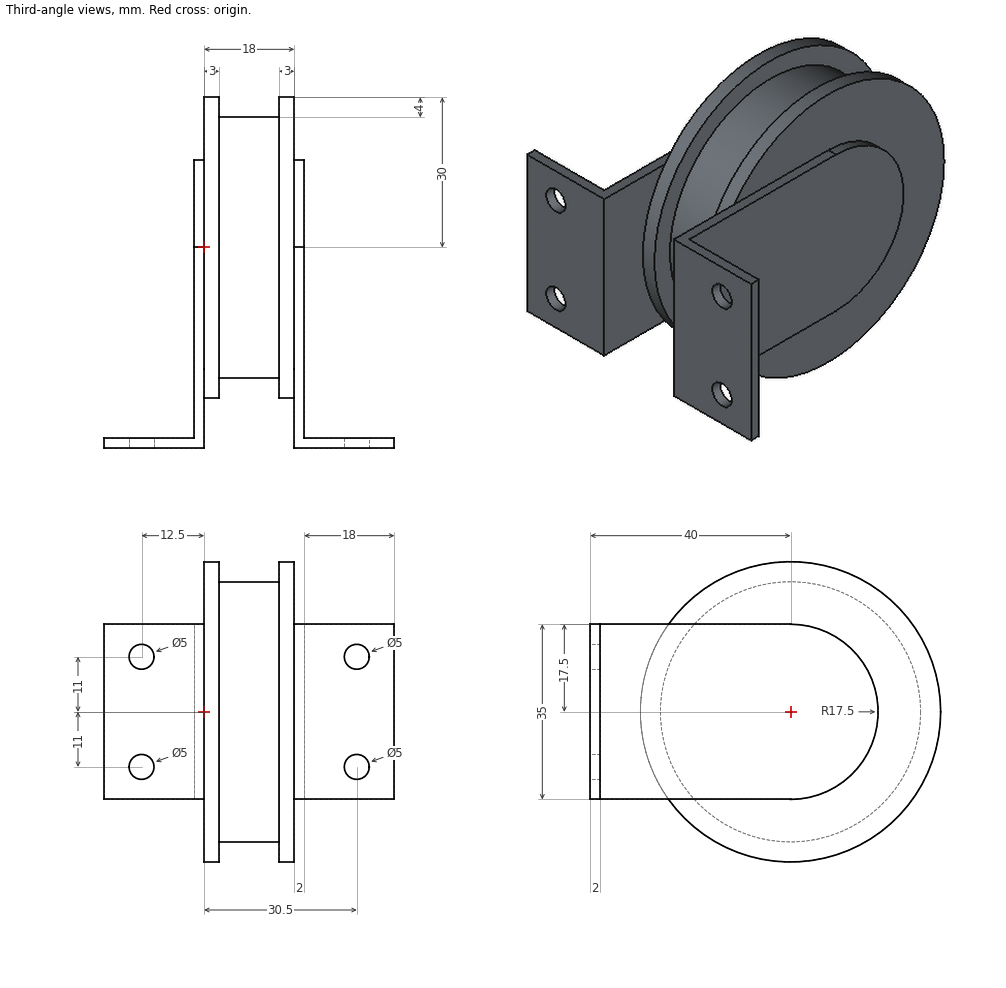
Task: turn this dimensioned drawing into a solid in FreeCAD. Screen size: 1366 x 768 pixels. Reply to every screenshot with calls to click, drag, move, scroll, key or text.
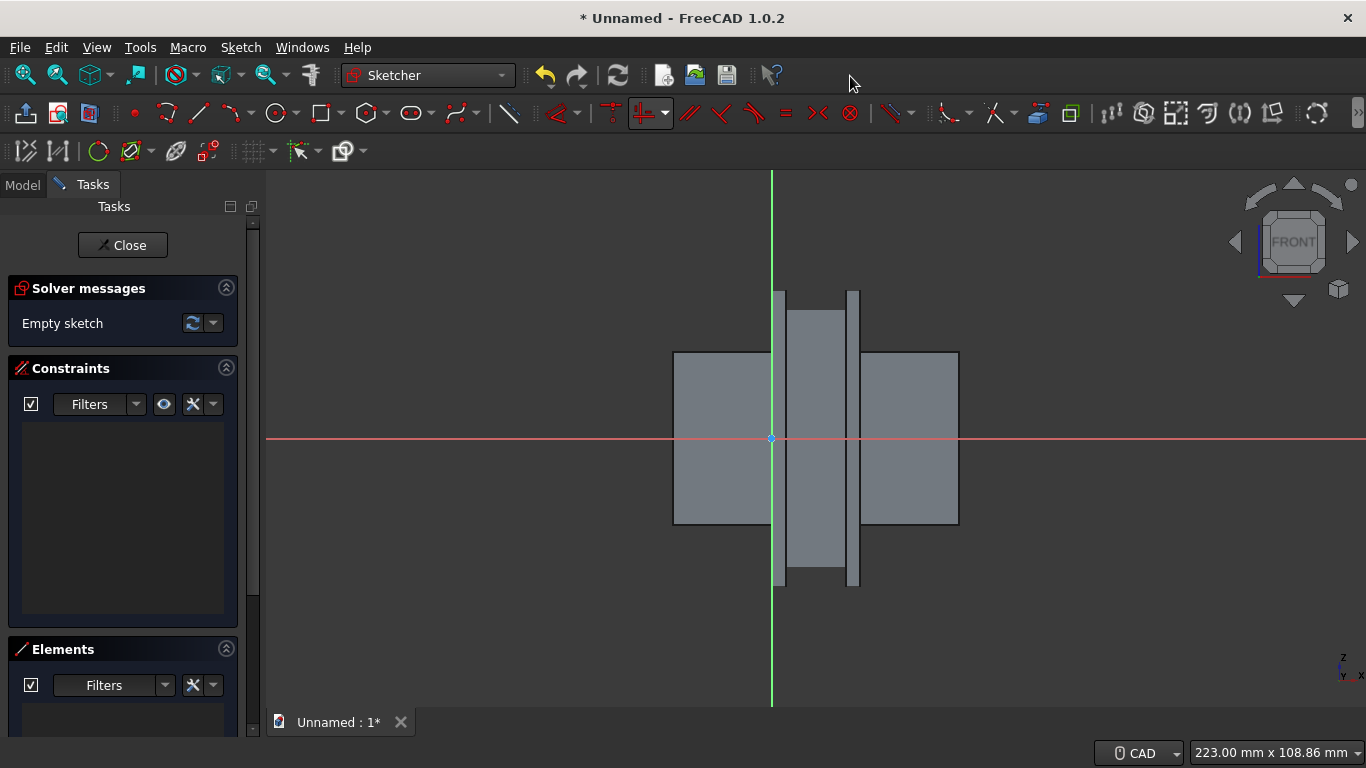
scroll(707, 380, up, 13)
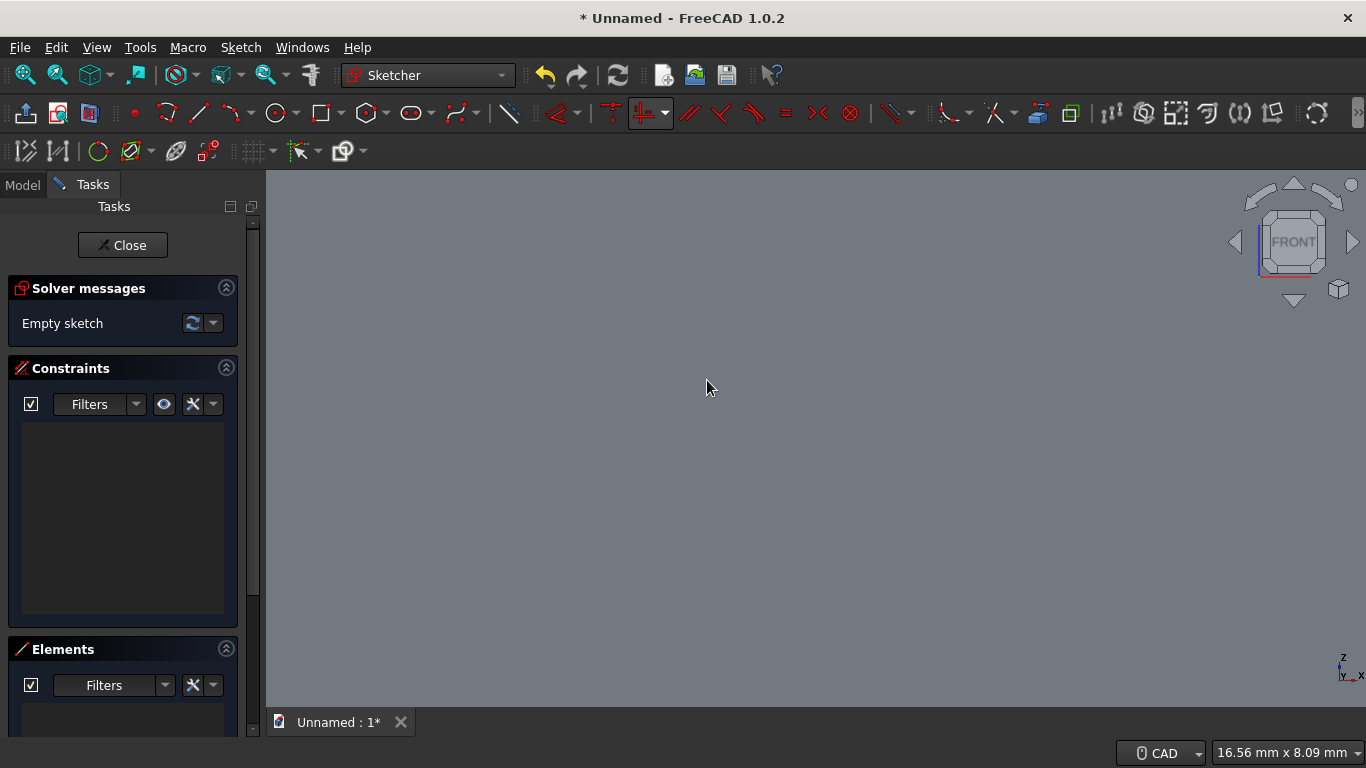
click(276, 114)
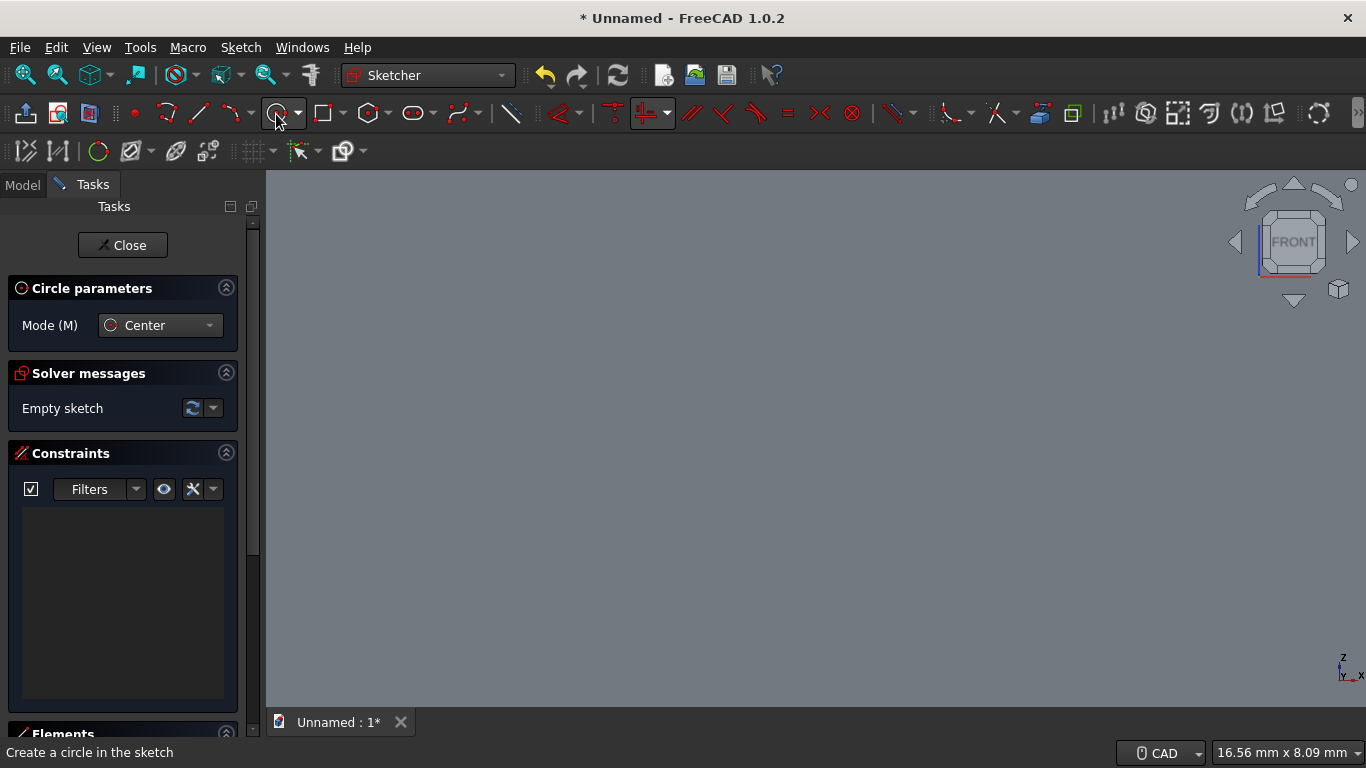
click(742, 432)
click(859, 315)
key(Escape)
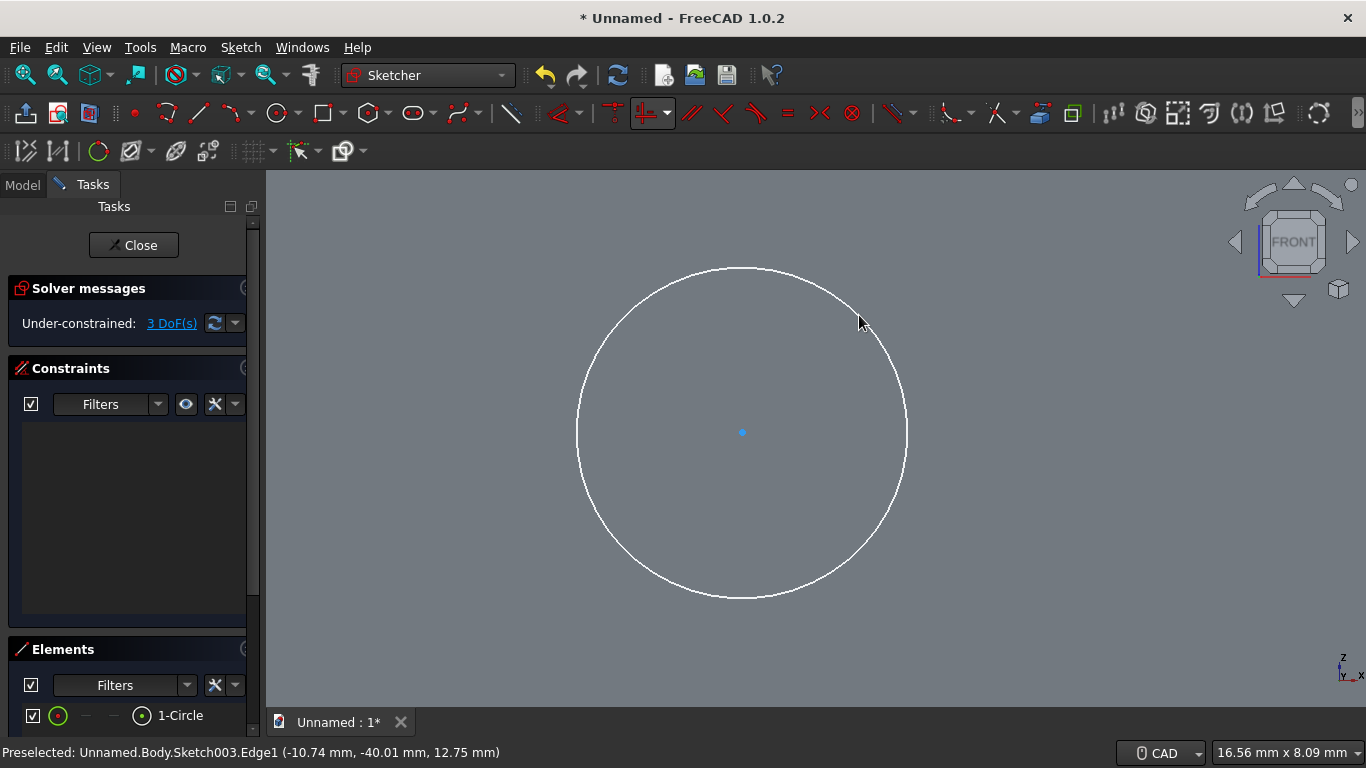
key(d)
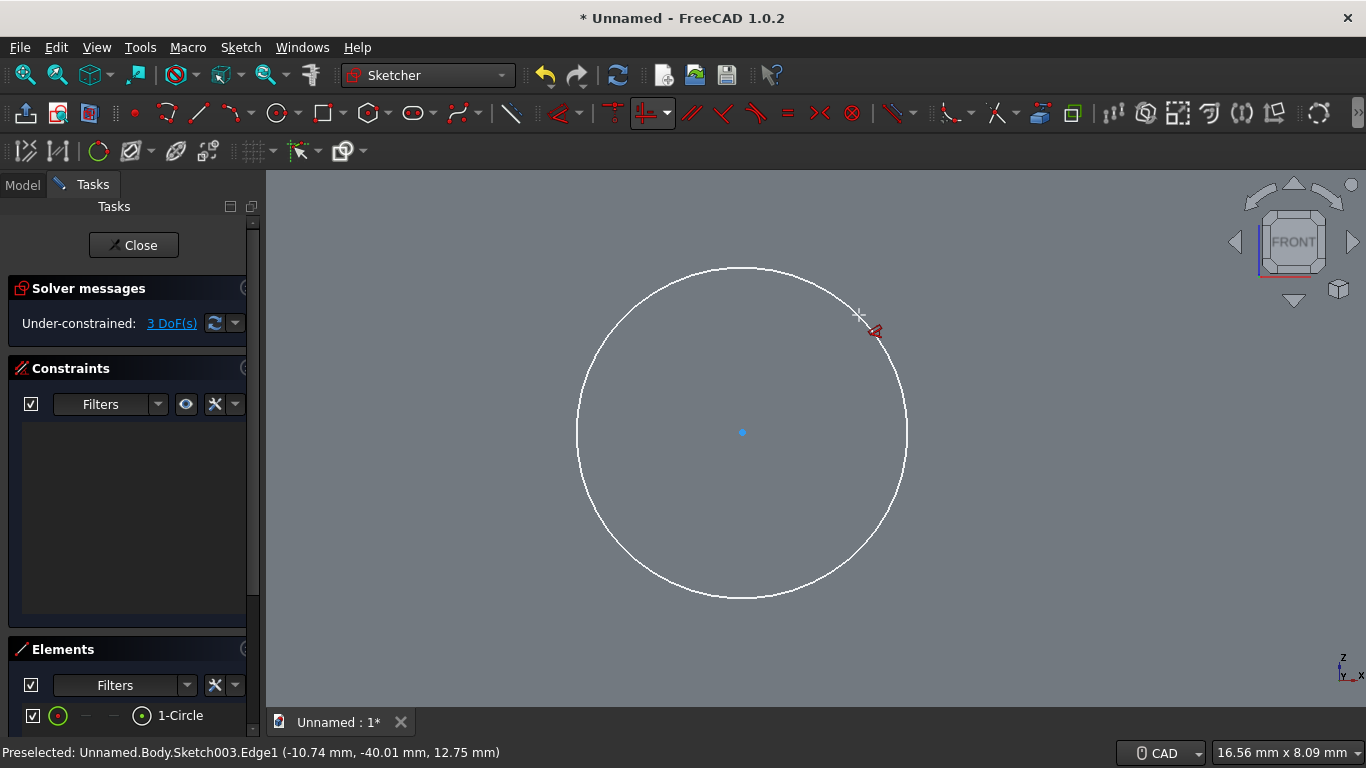
click(859, 316)
click(882, 293)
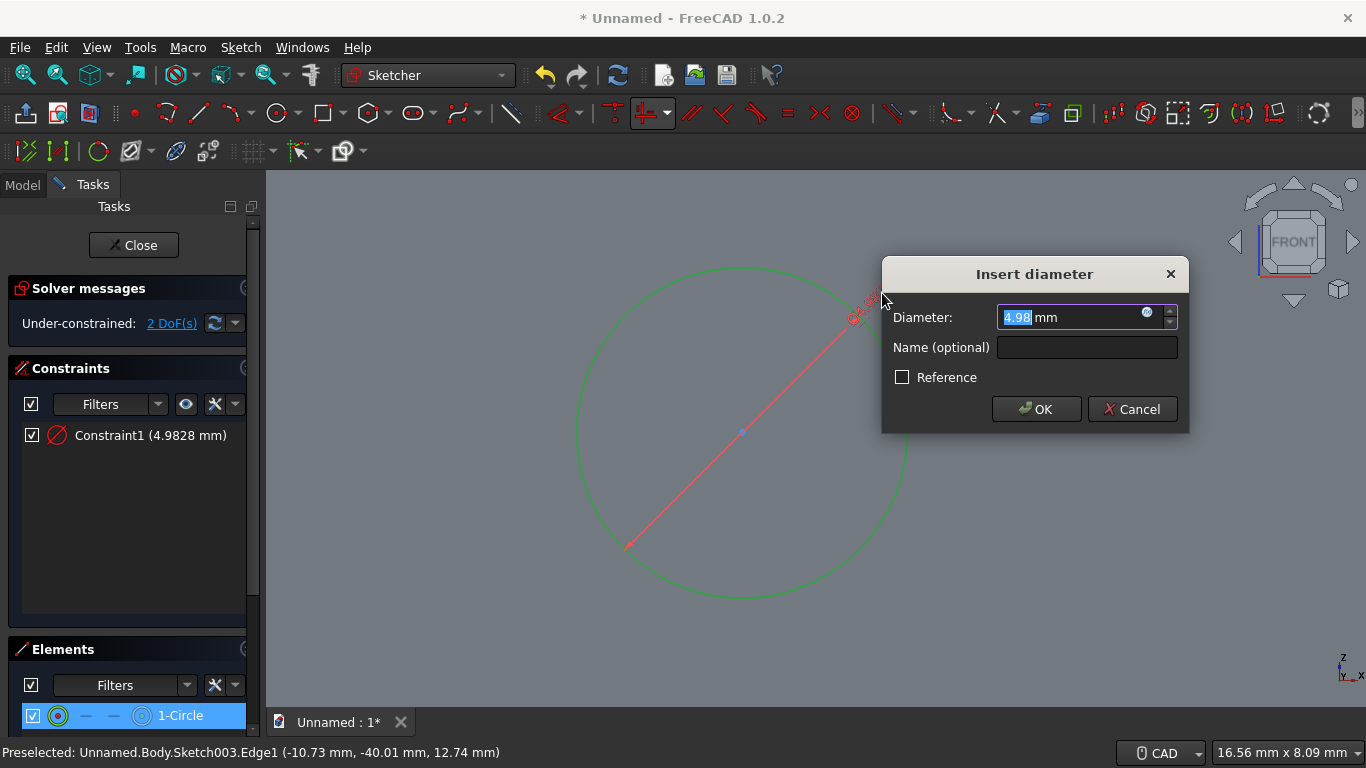
text(5)
key(Return)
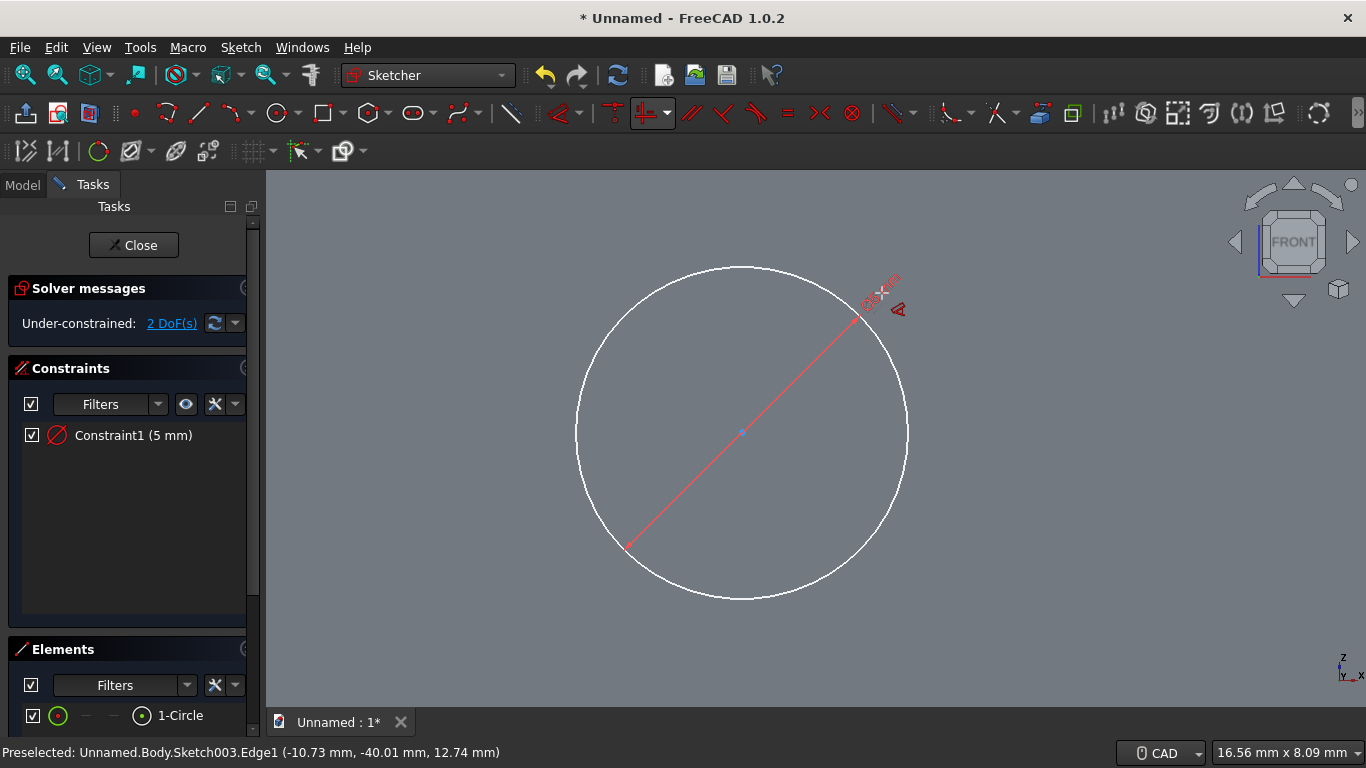
click(742, 433)
click(708, 556)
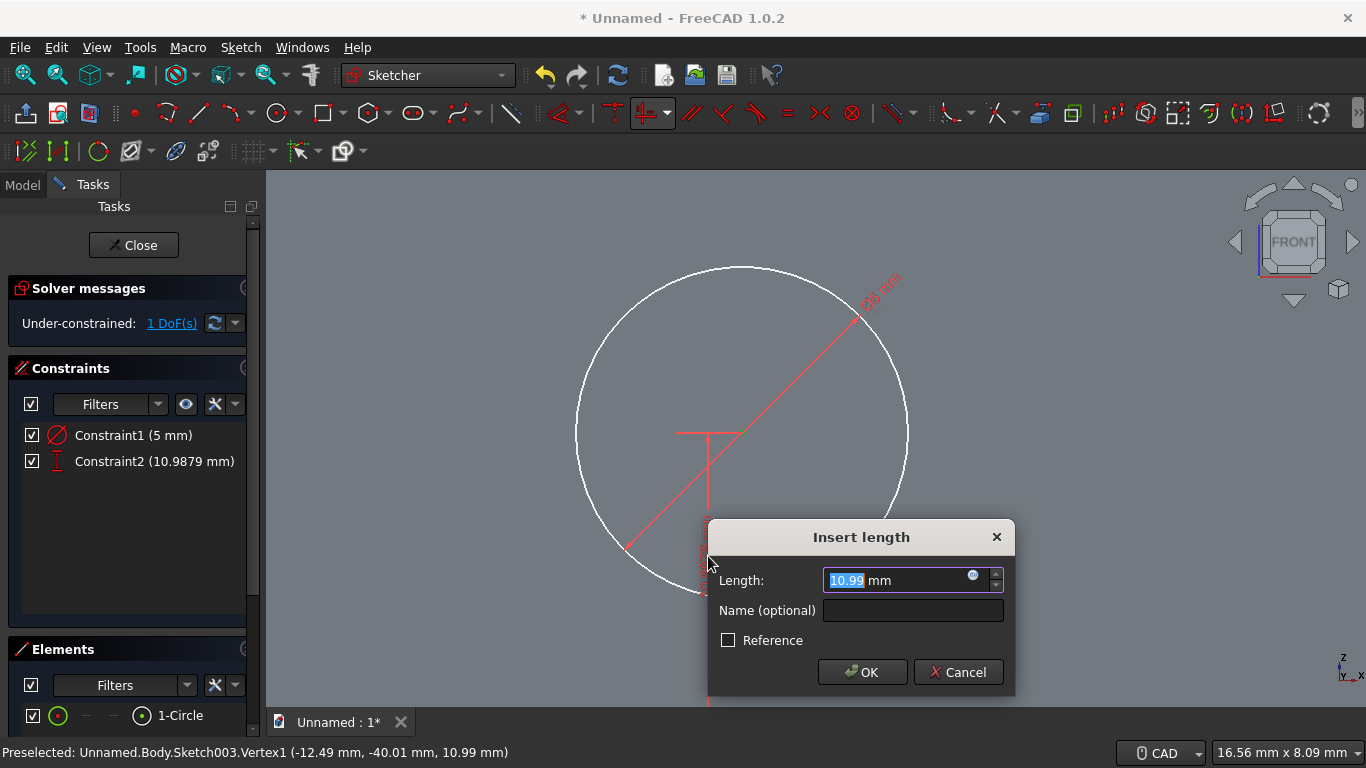
text(11)
key(Return)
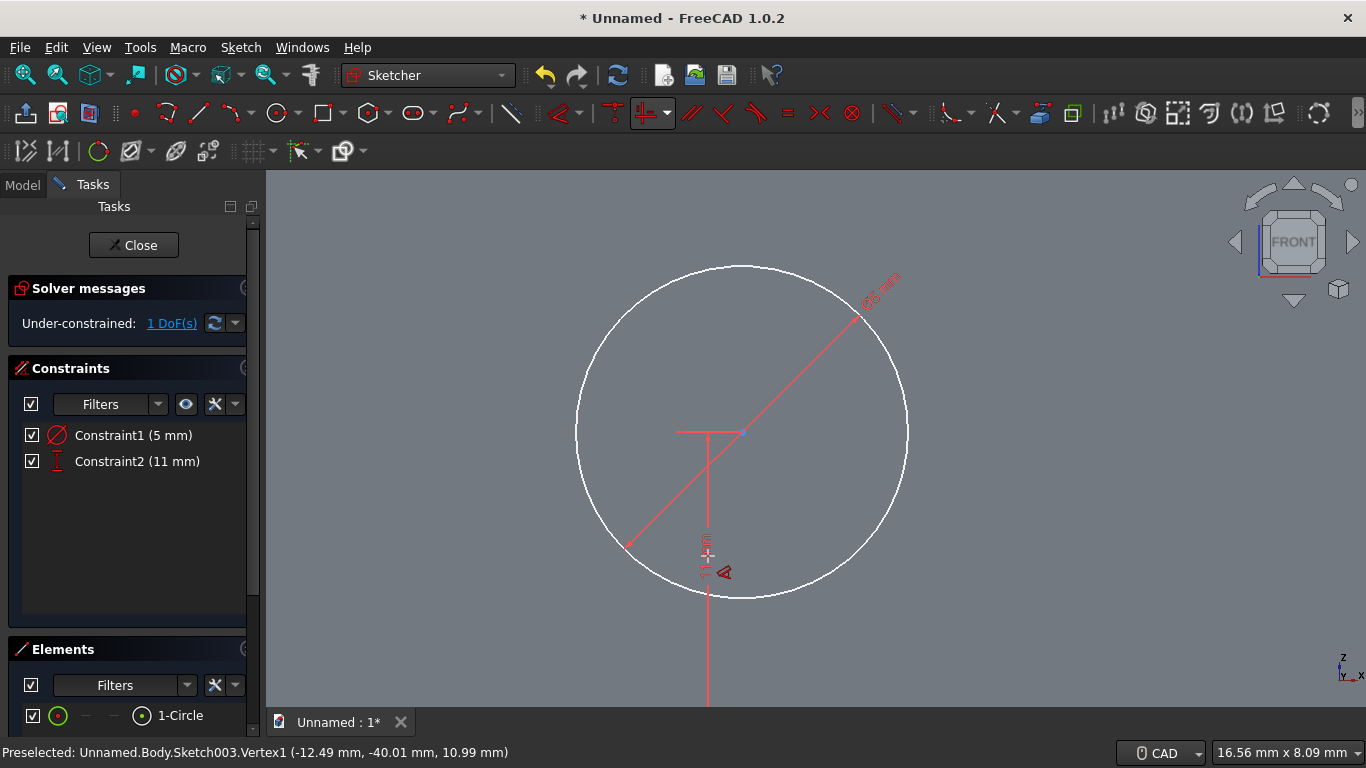
click(742, 432)
click(971, 398)